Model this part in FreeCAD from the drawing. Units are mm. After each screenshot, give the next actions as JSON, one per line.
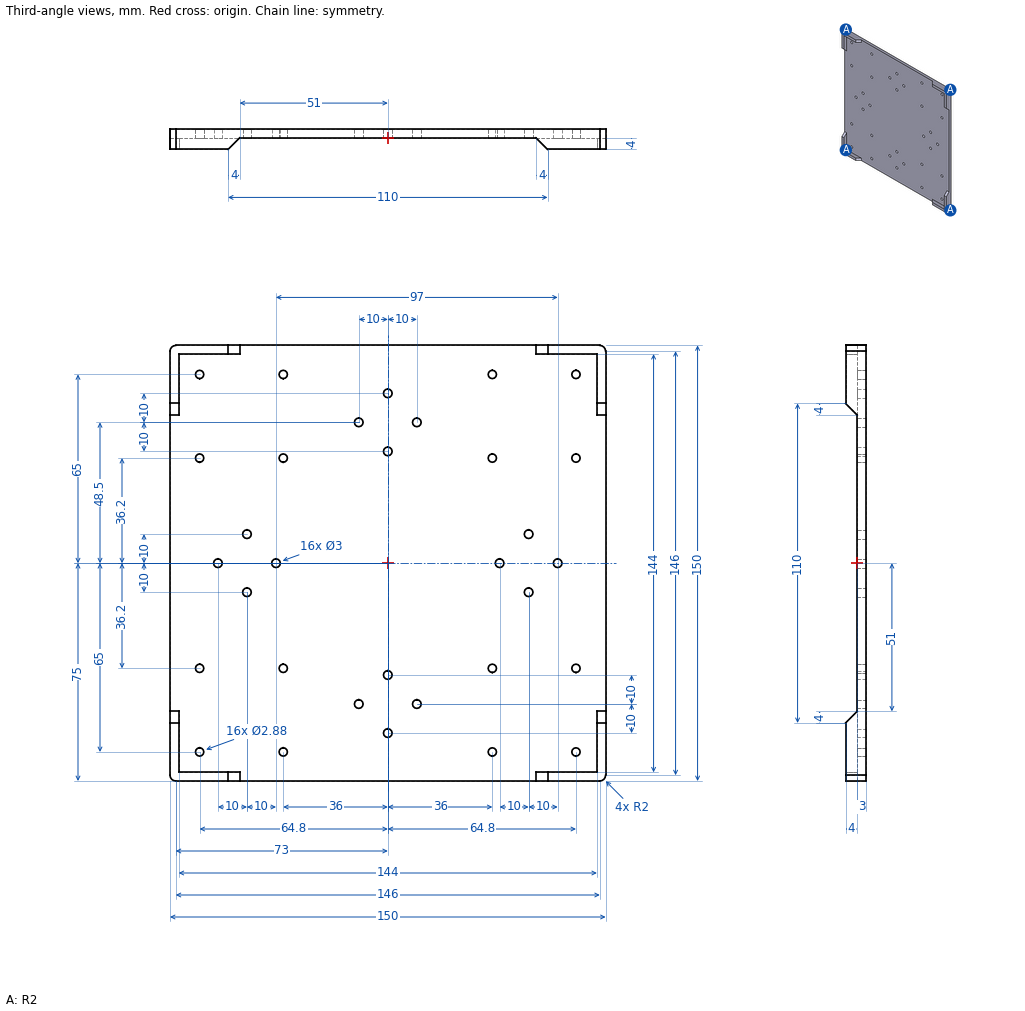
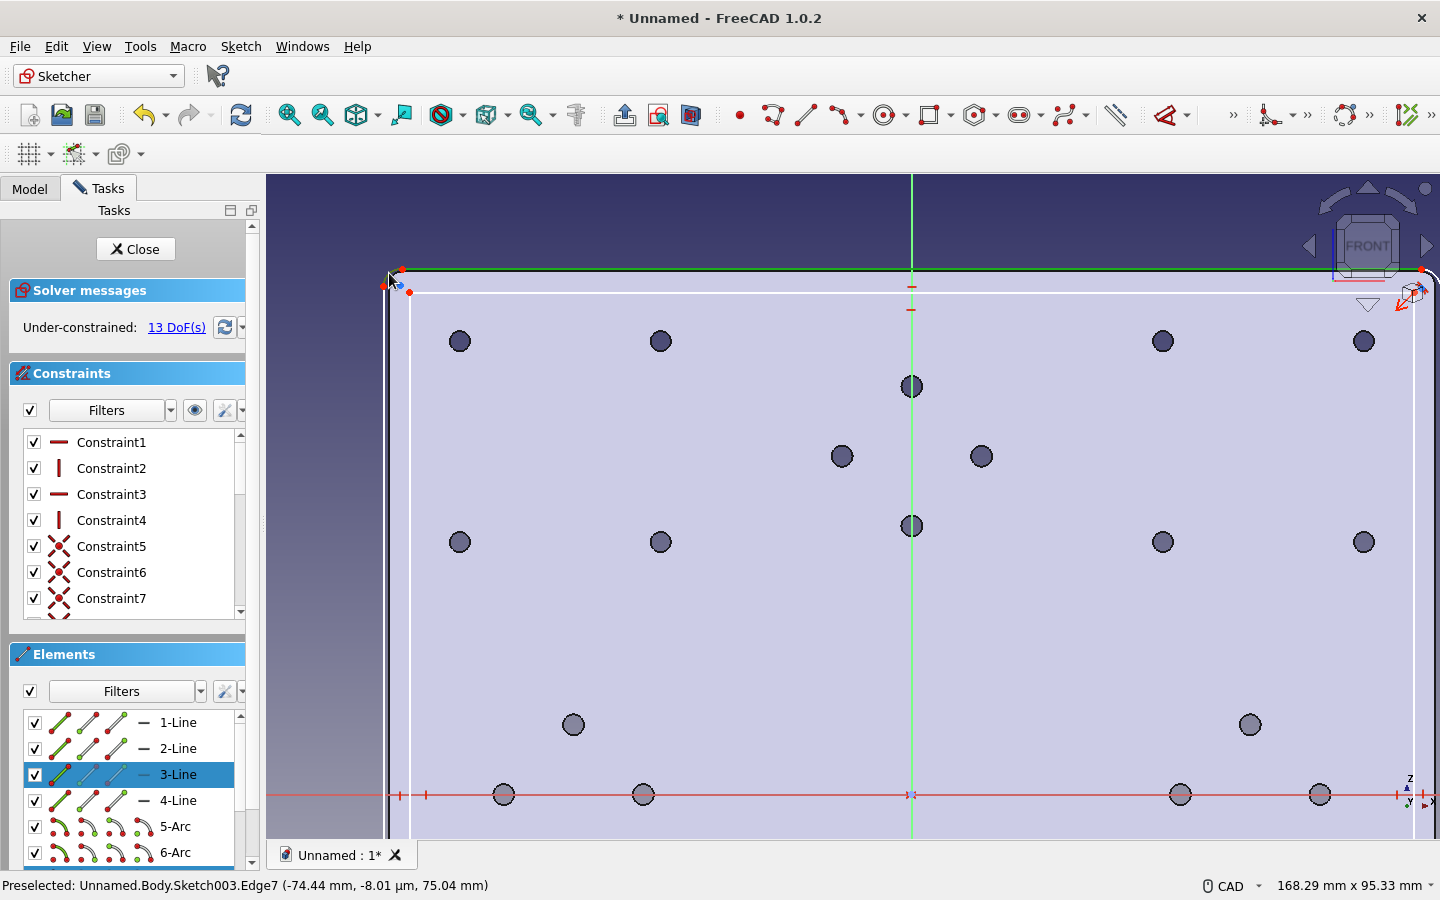
{"action": "key", "text": "t"}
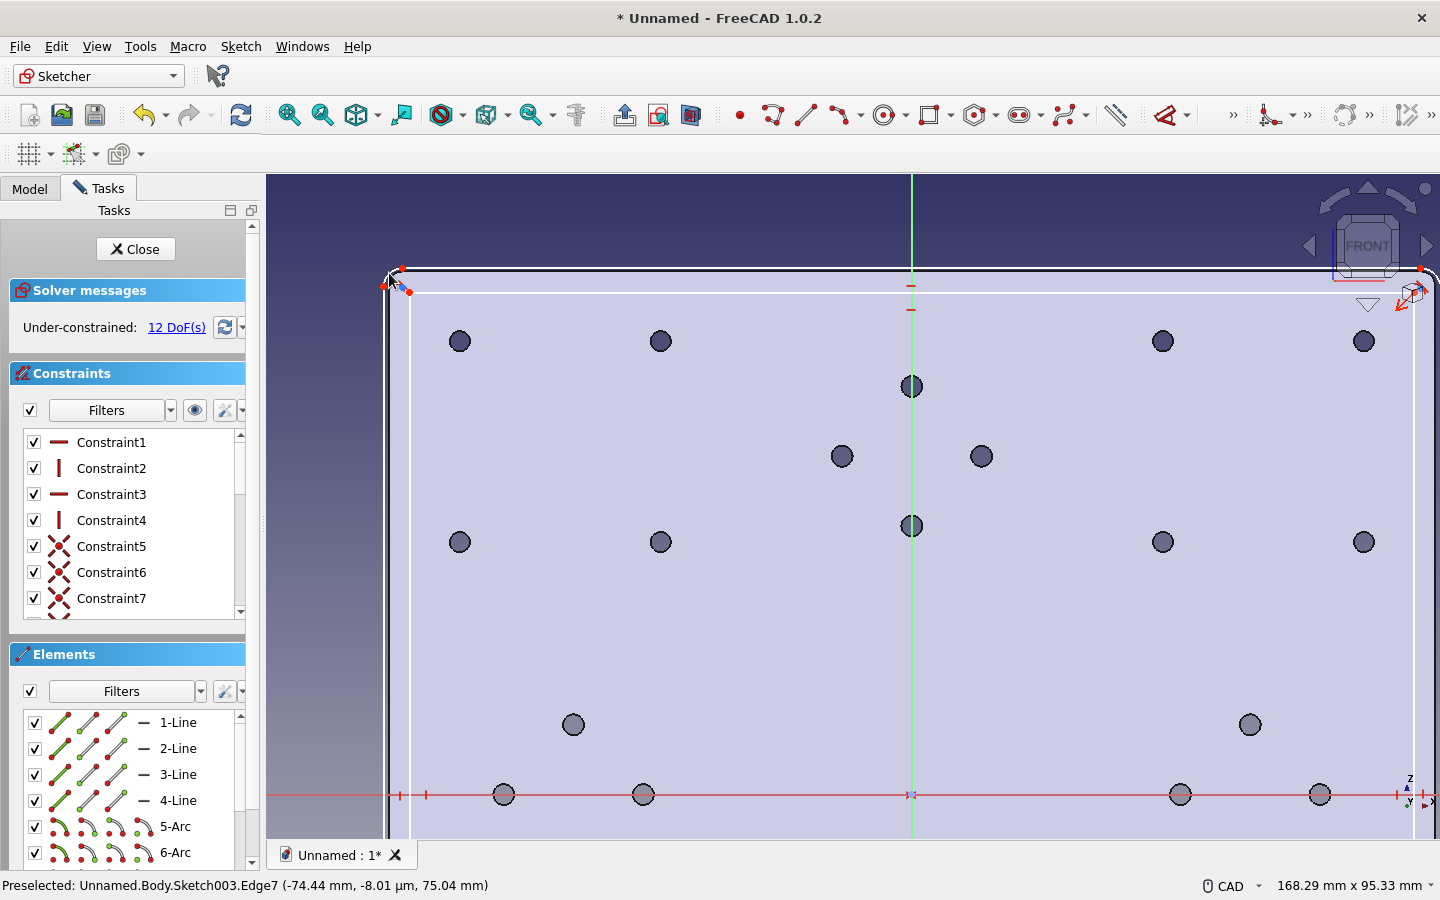
{"action": "left_click", "coordinate": [384, 592]}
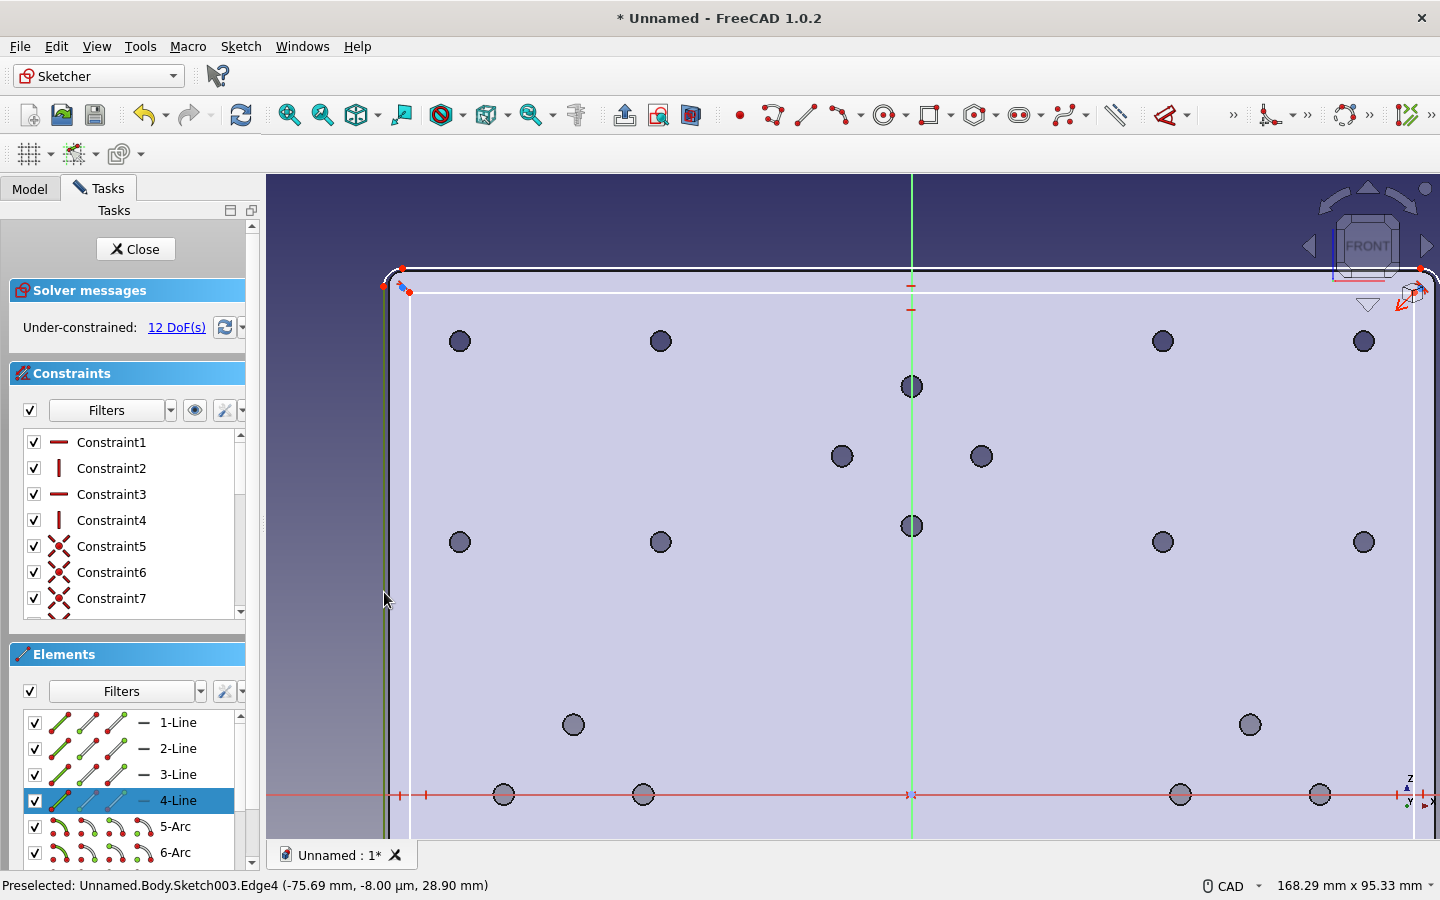
{"action": "left_click", "coordinate": [390, 274]}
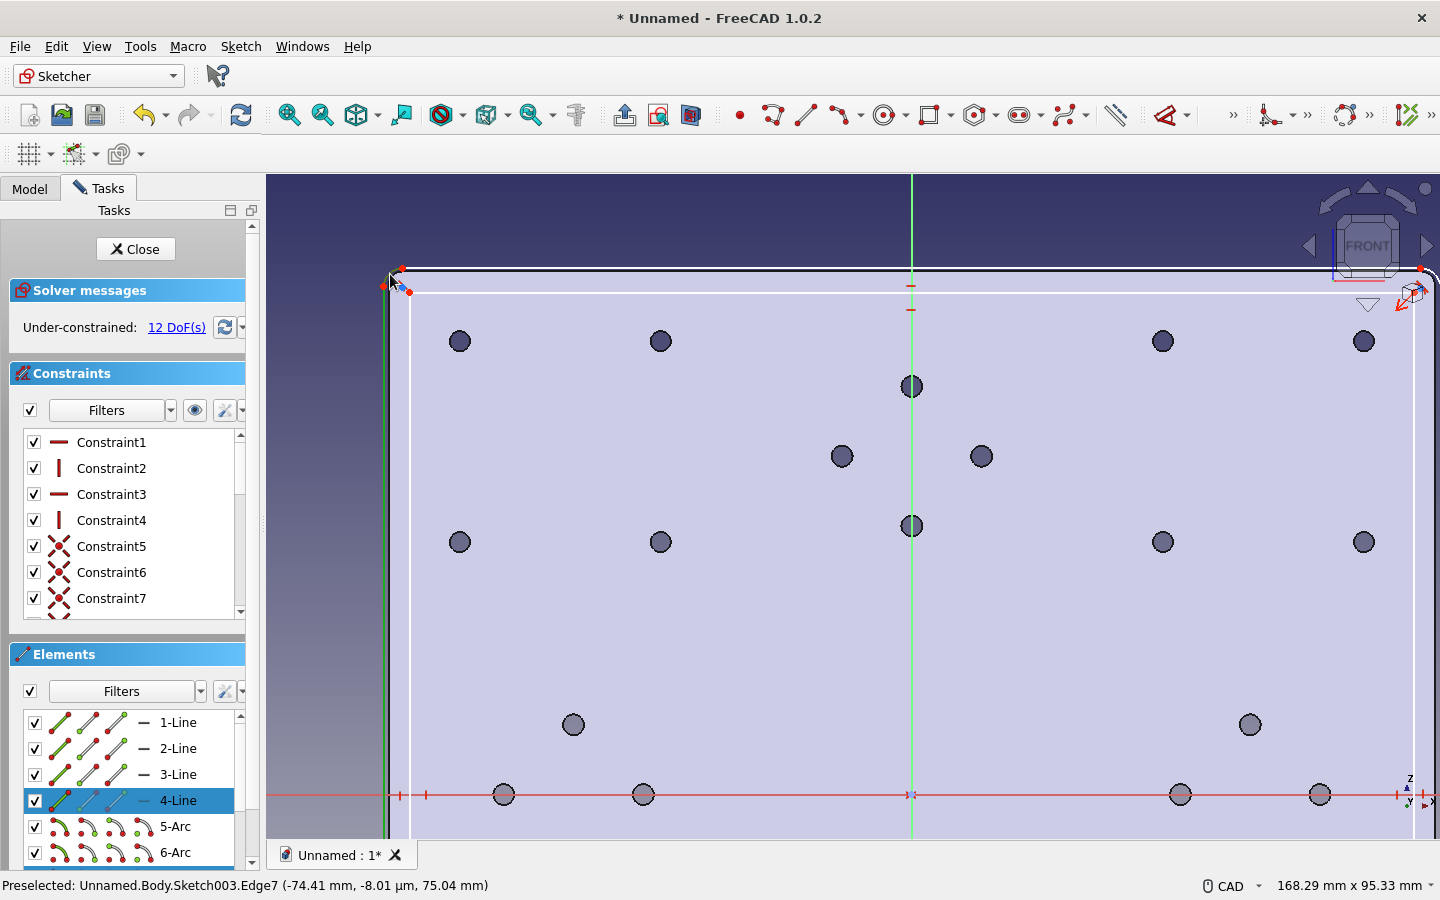
{"action": "key", "text": "t"}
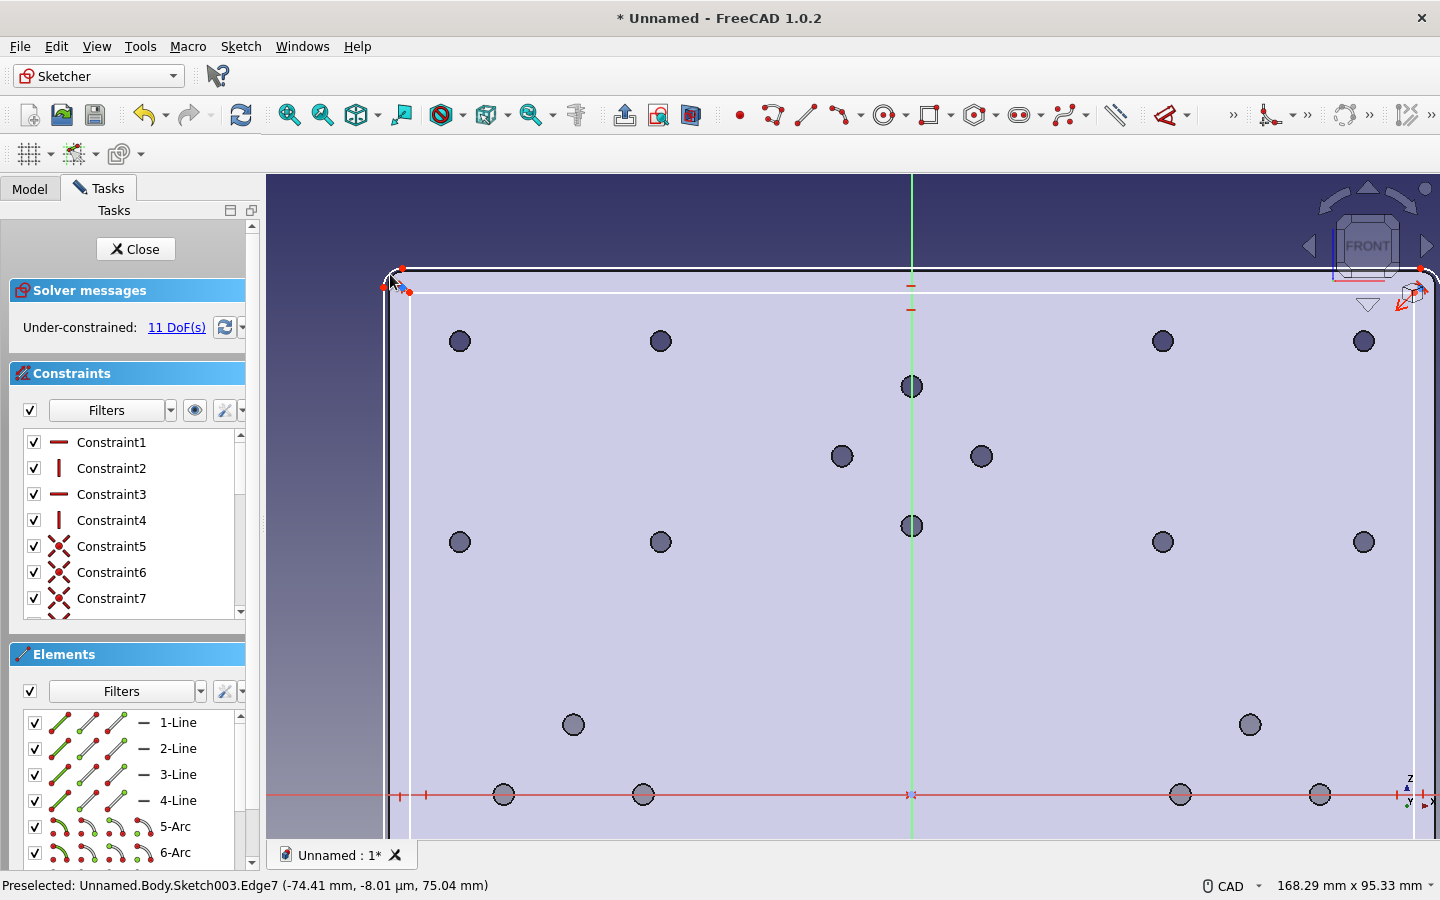
{"action": "left_click", "coordinate": [384, 592]}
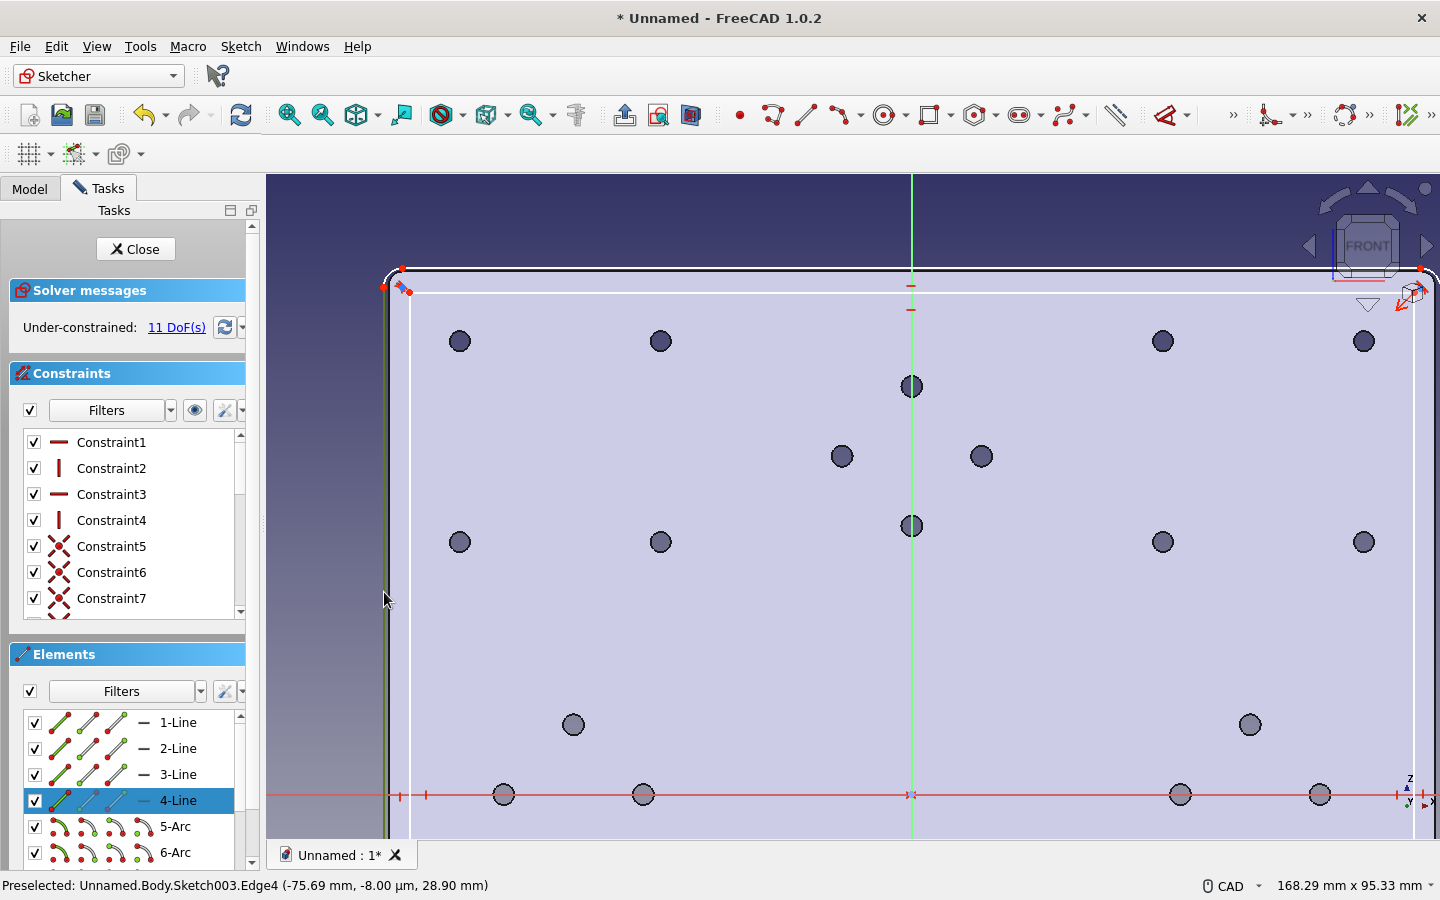
{"action": "scroll", "coordinate": [681, 271], "scroll_direction": "down", "scroll_amount": 4}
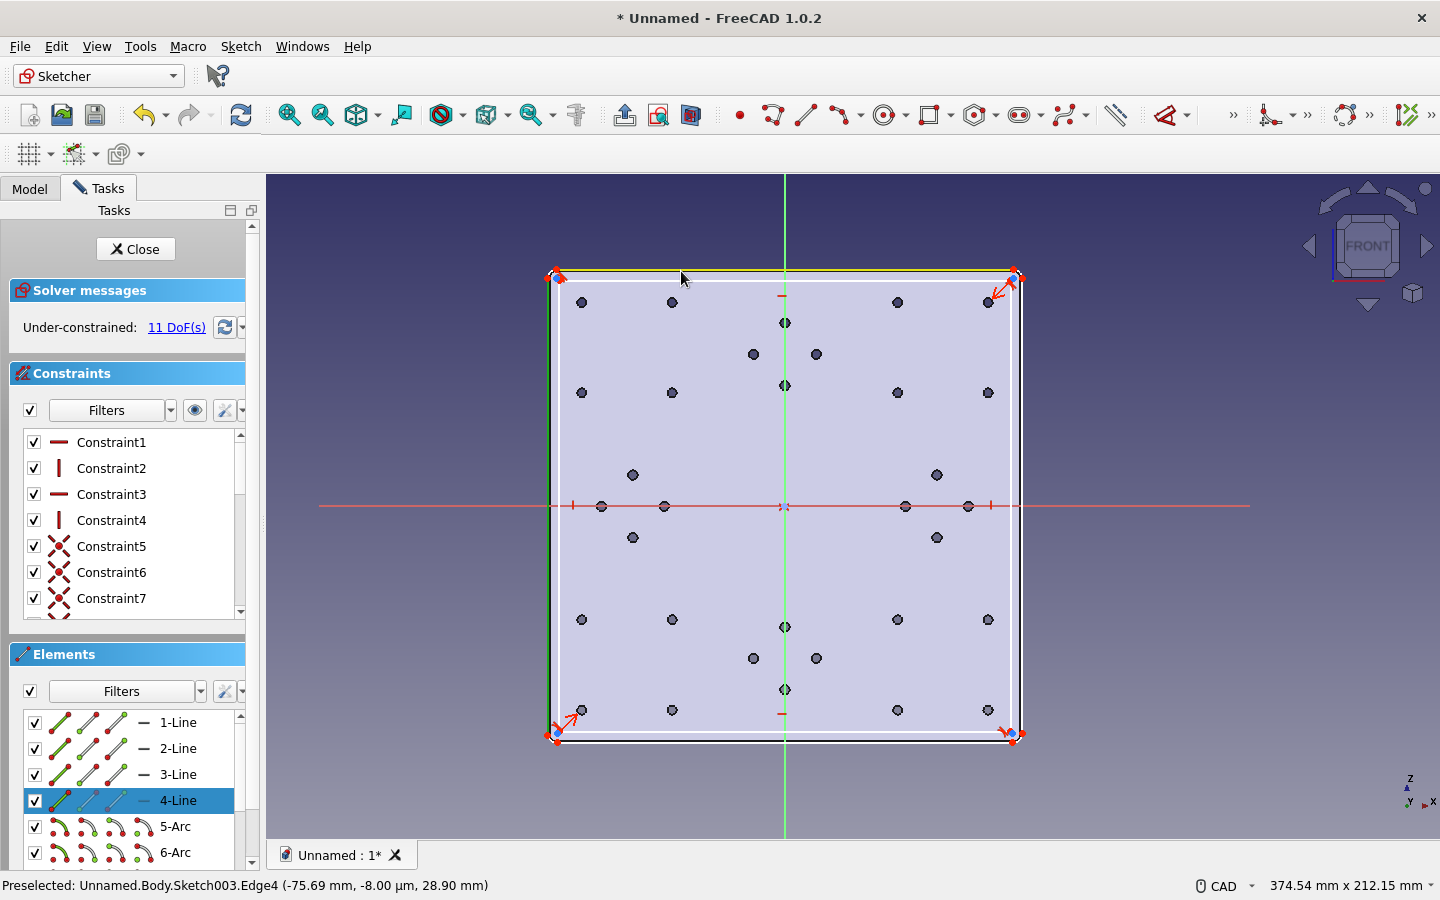
{"action": "scroll", "coordinate": [551, 741], "scroll_direction": "up", "scroll_amount": 5}